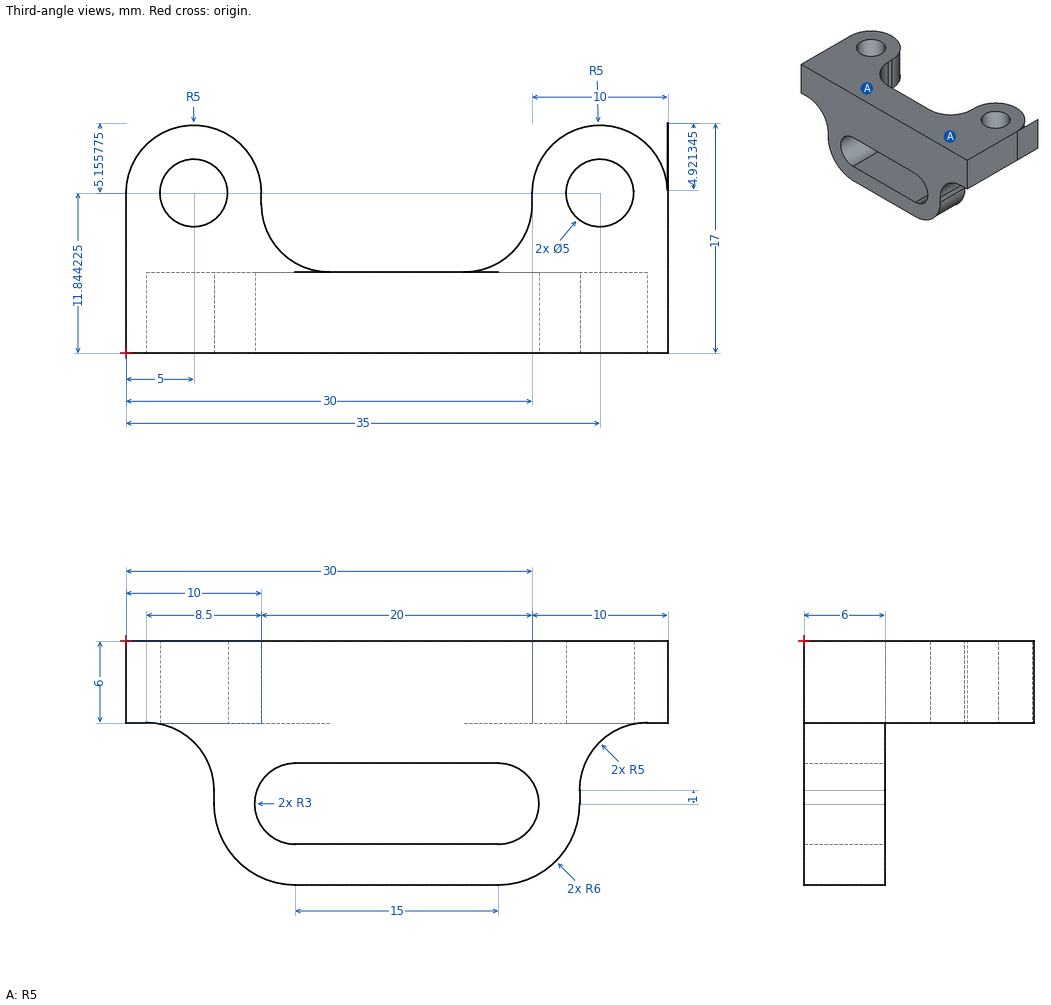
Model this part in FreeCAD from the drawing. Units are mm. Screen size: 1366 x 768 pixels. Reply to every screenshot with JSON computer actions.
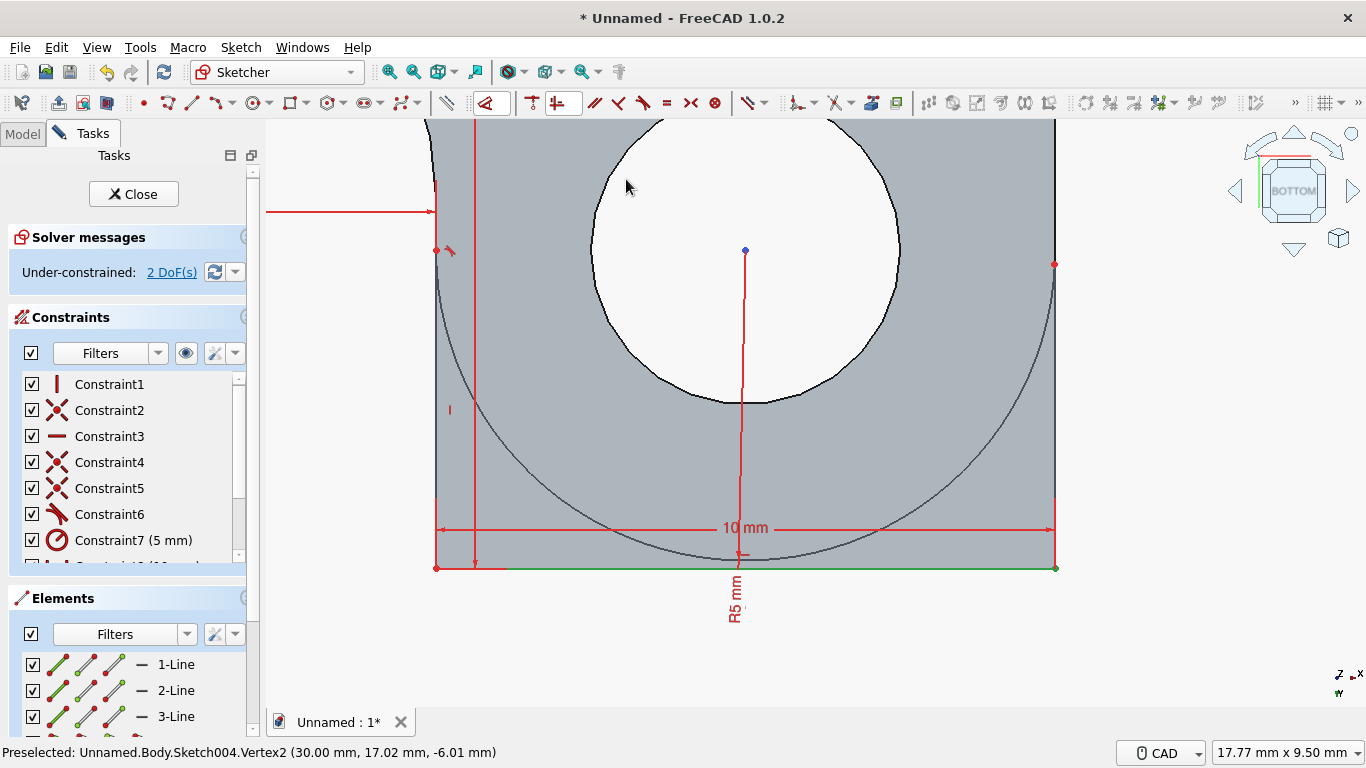
{"action": "left_click", "coordinate": [436, 346]}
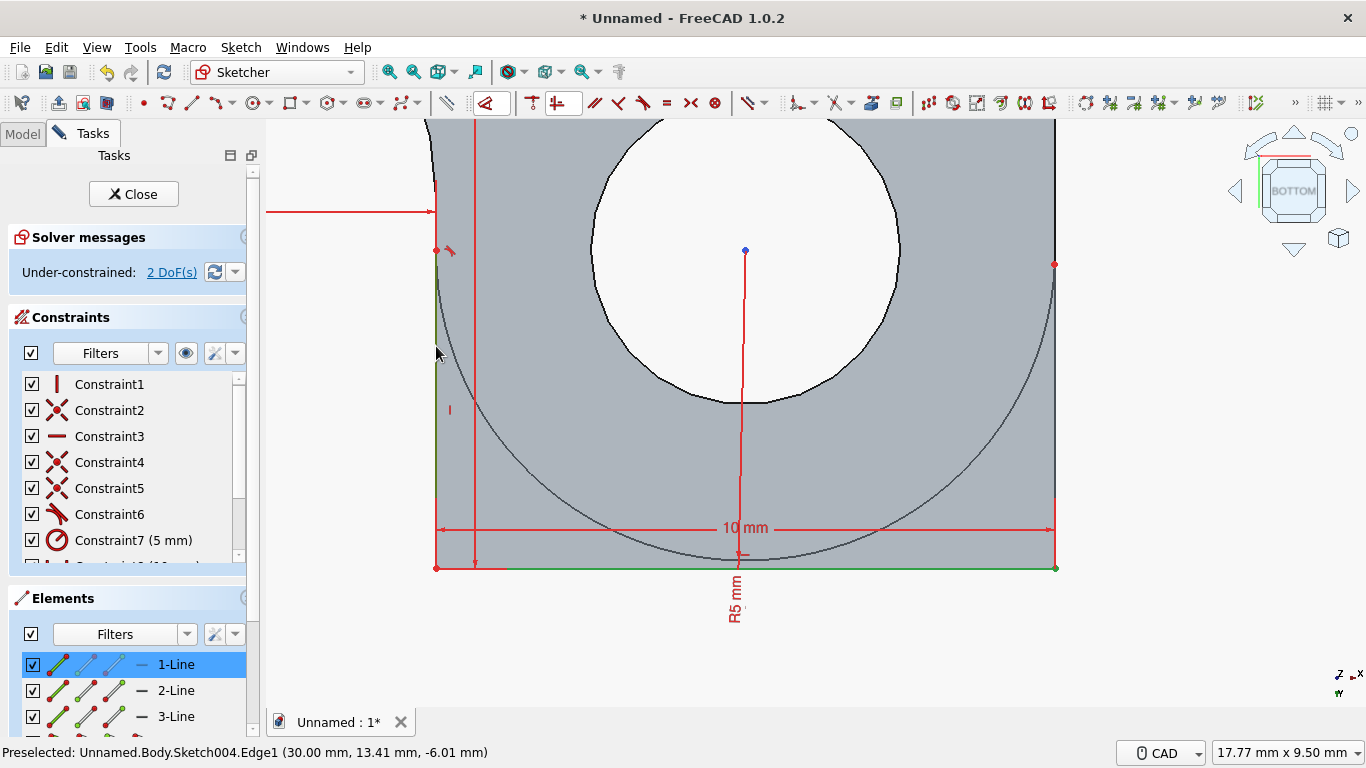
{"action": "left_click", "coordinate": [504, 104]}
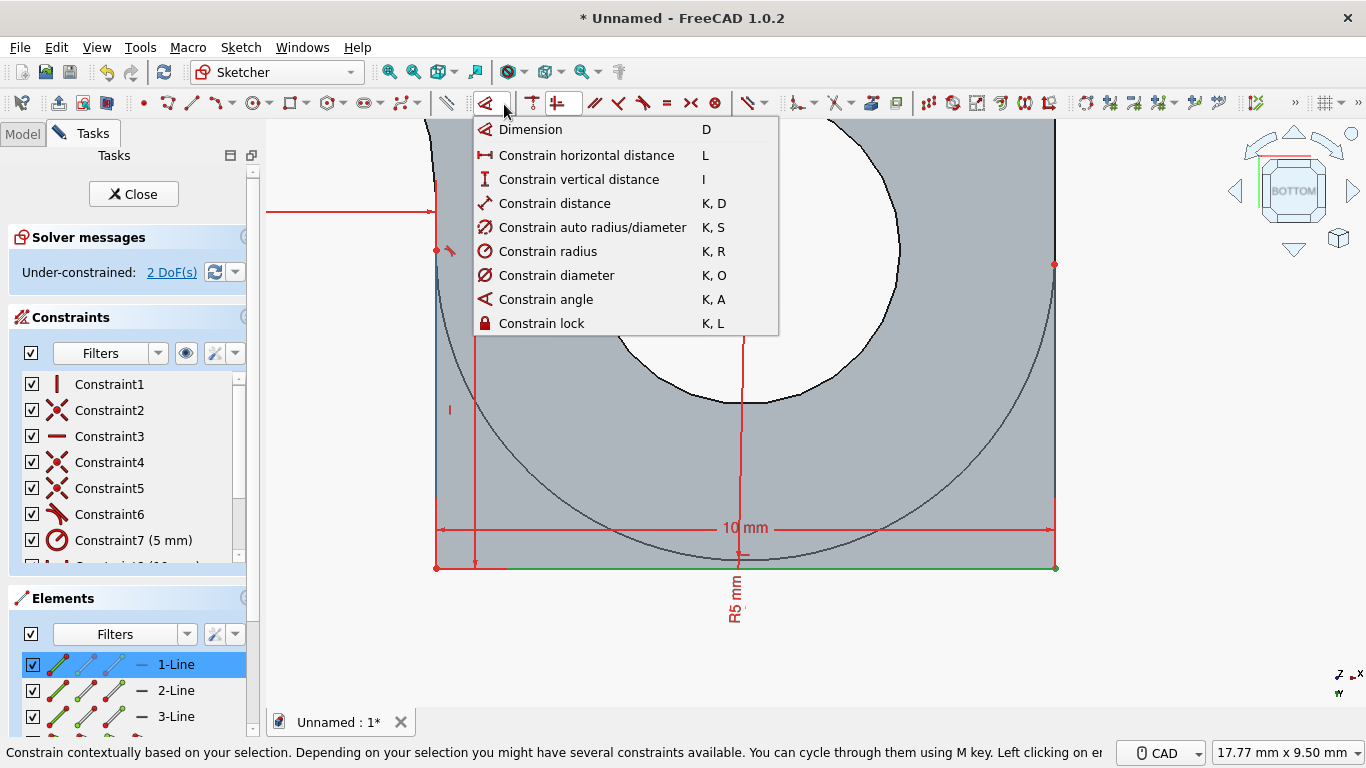
{"action": "left_click", "coordinate": [626, 179]}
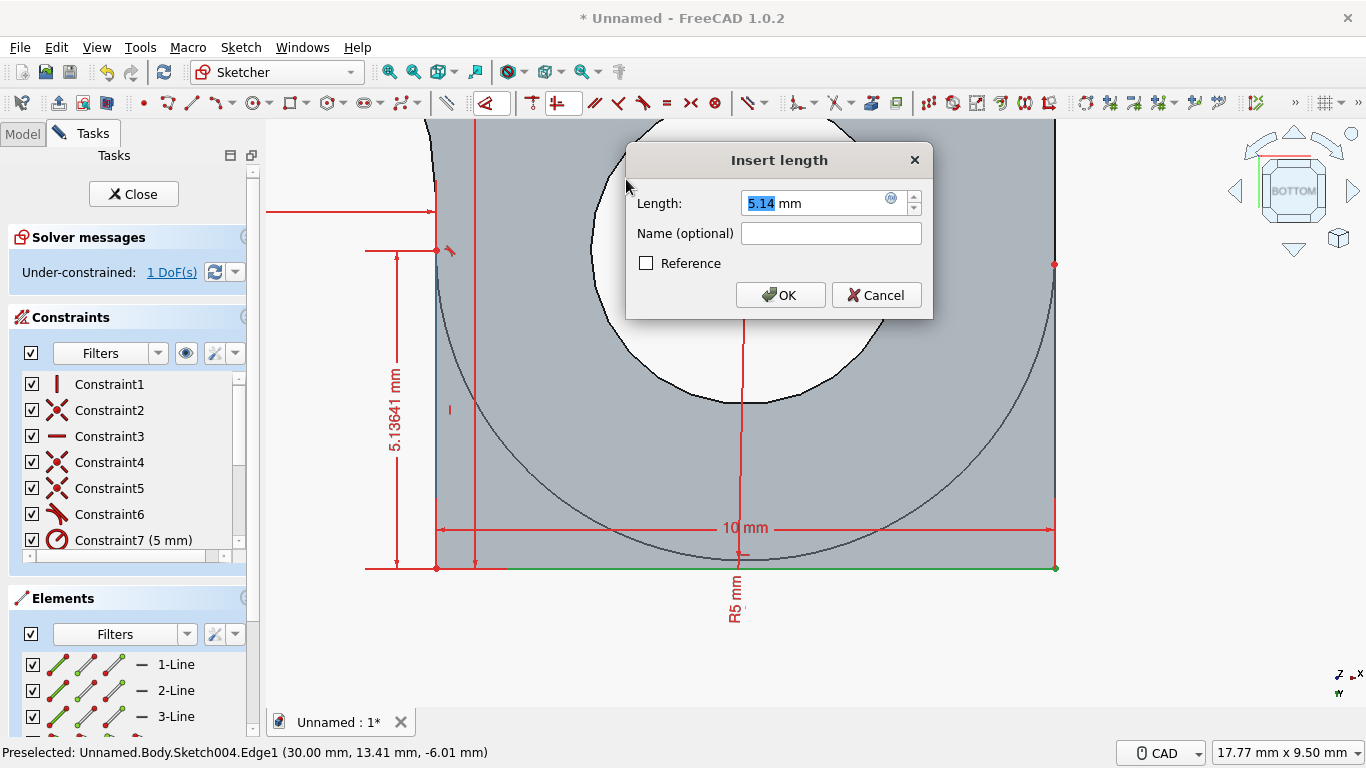
{"action": "type", "text": "5.155775"}
{"action": "key", "text": "Return"}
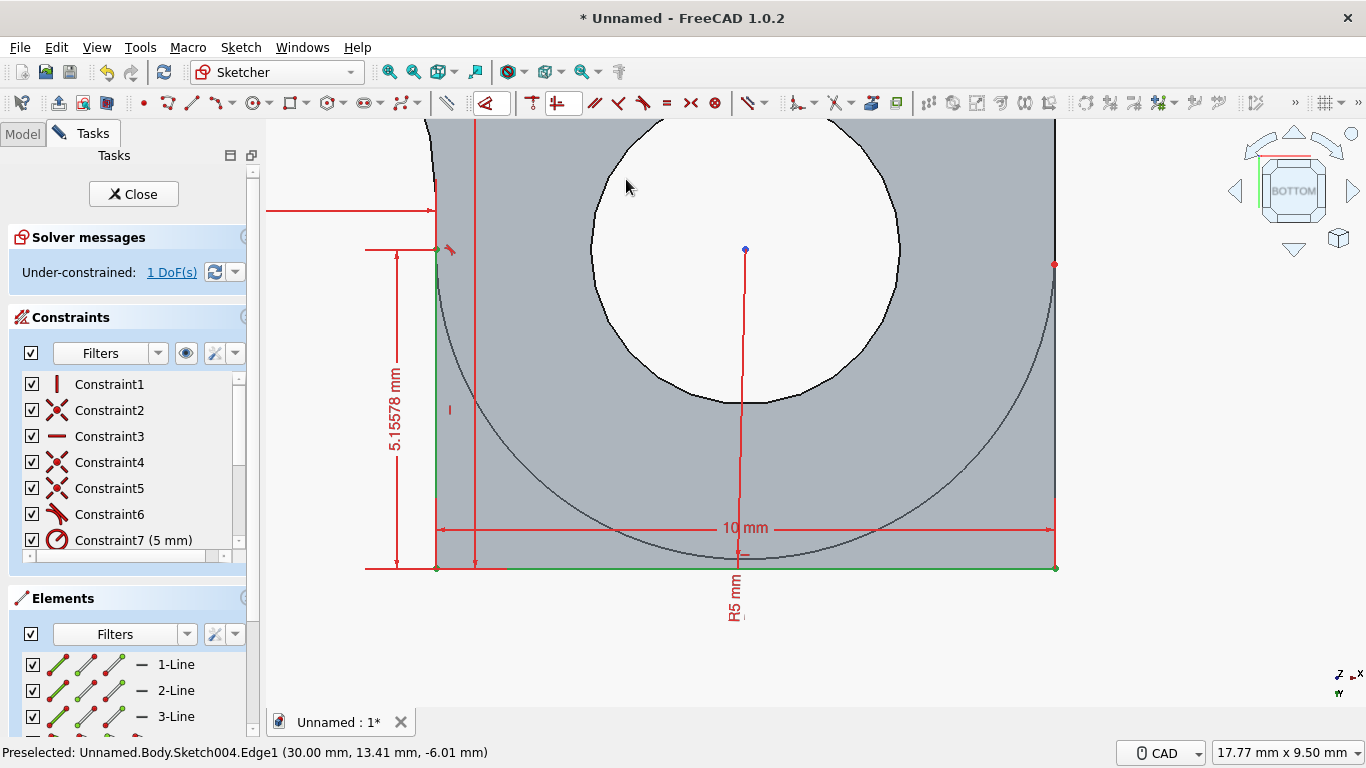
{"action": "left_click", "coordinate": [1055, 478]}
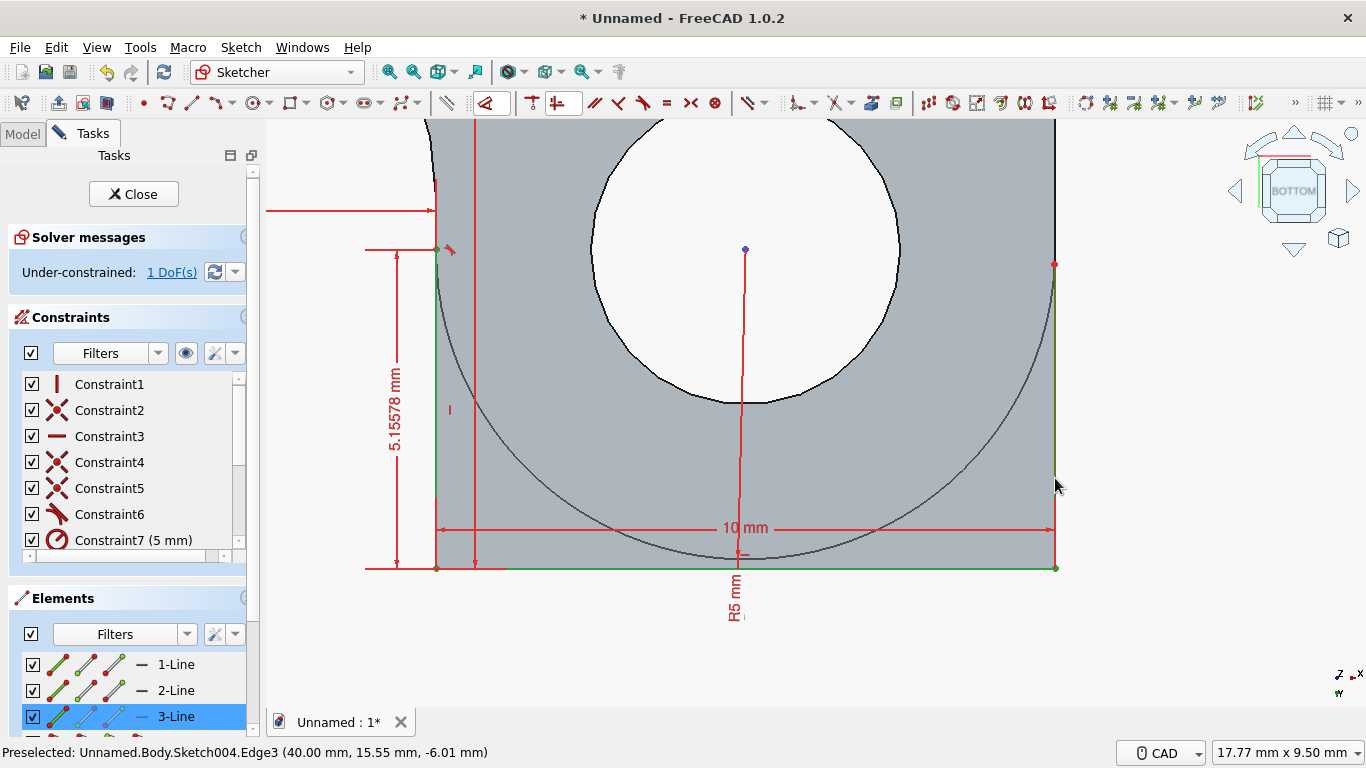
{"action": "key", "text": "i"}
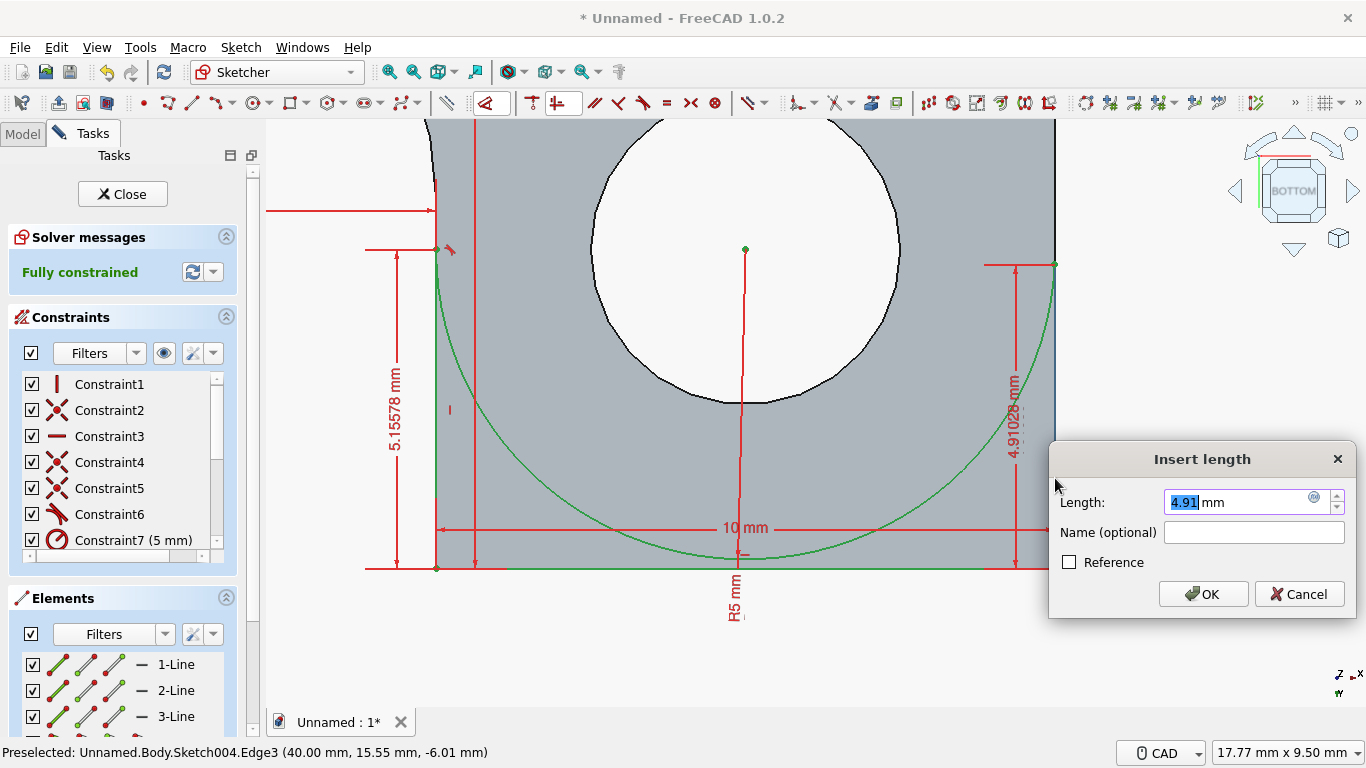
{"action": "type", "text": "4.921345"}
{"action": "key", "text": "Return"}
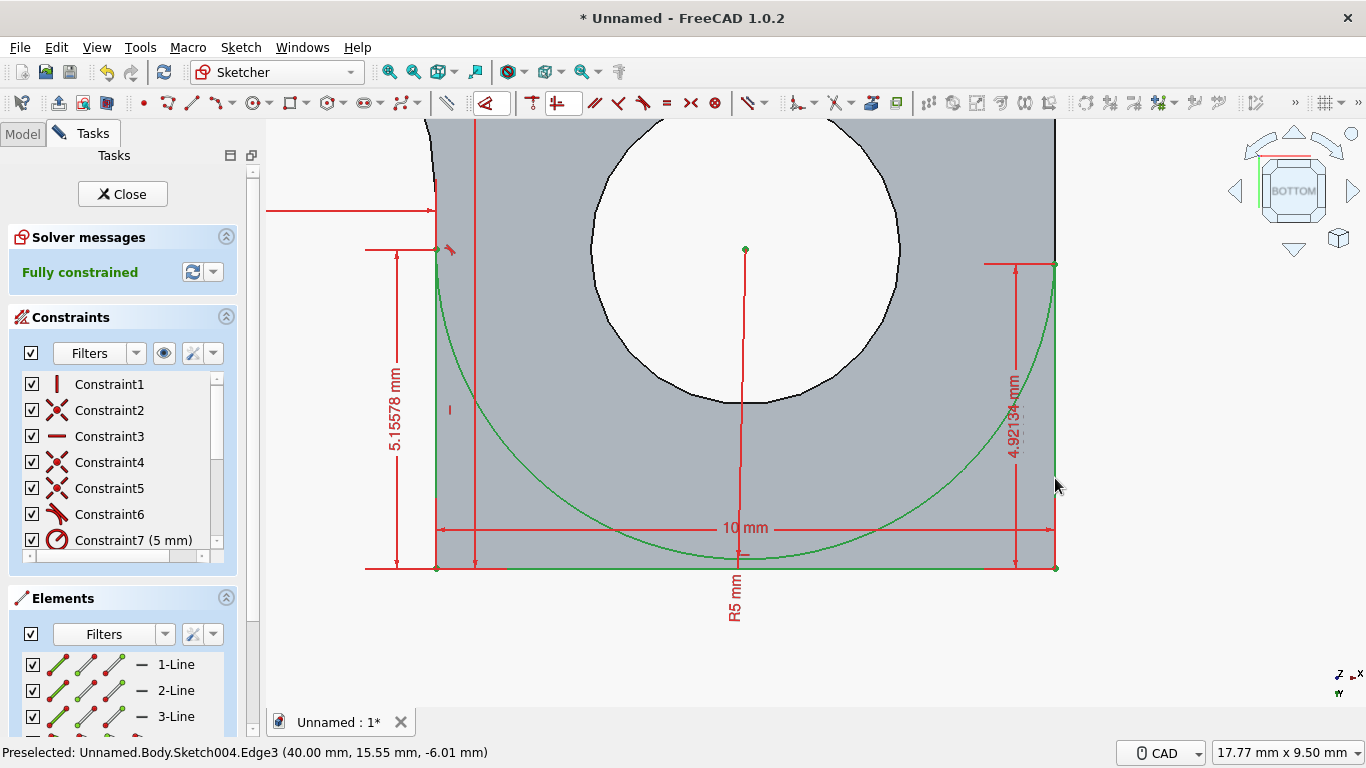
{"action": "left_click", "coordinate": [123, 194]}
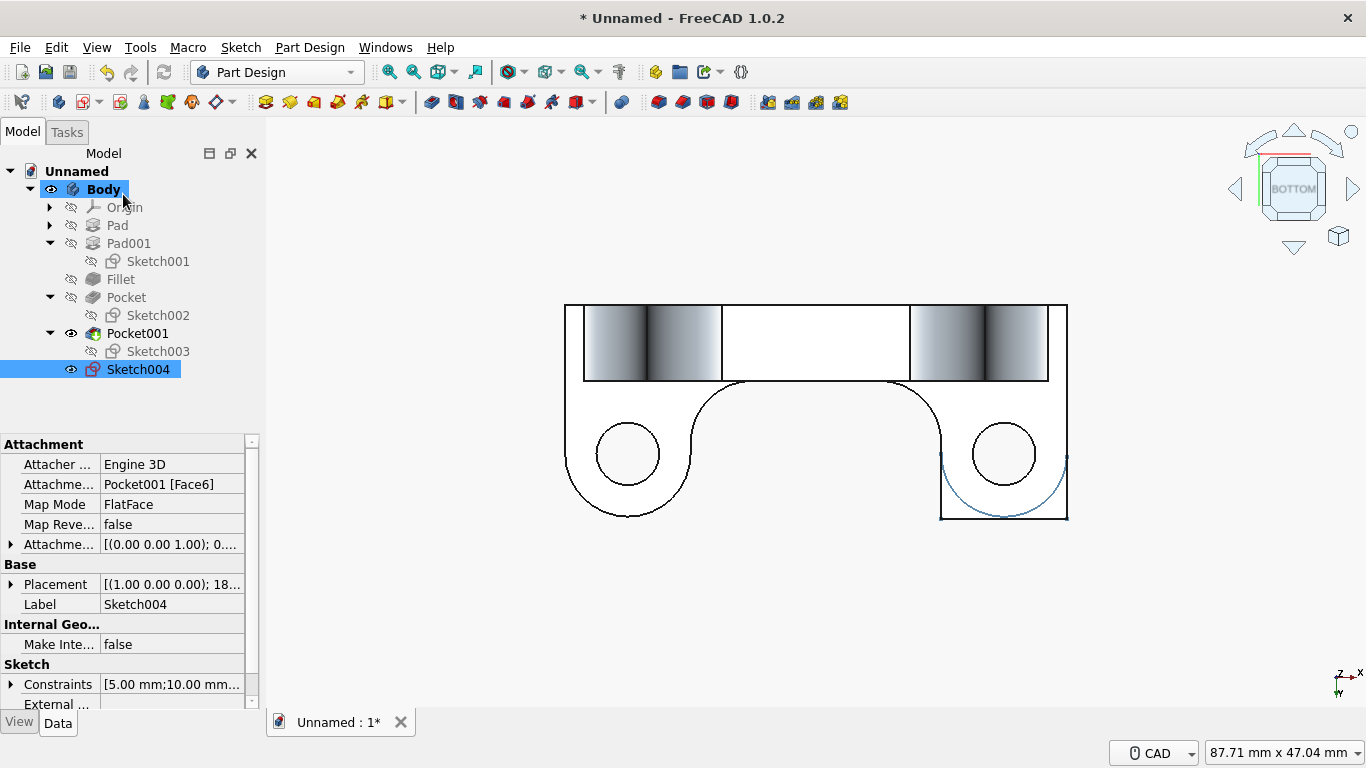
{"action": "left_click", "coordinate": [432, 102]}